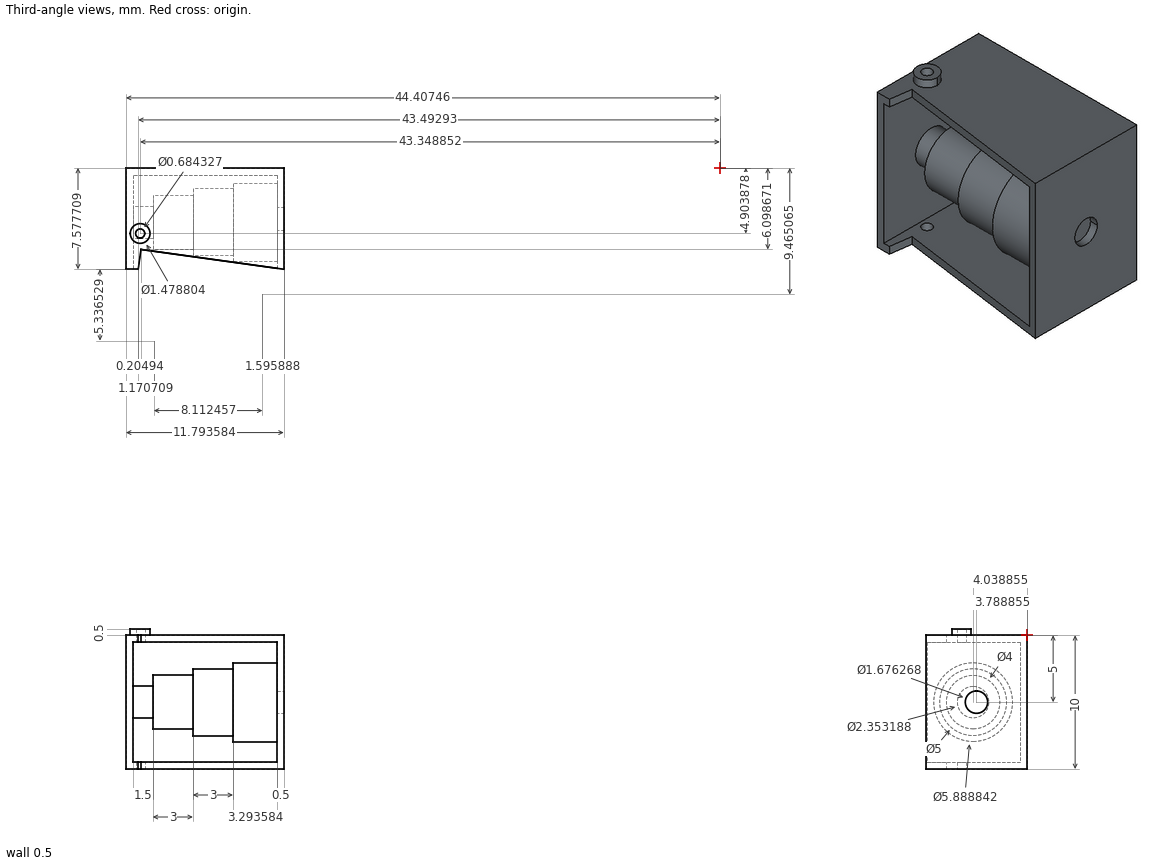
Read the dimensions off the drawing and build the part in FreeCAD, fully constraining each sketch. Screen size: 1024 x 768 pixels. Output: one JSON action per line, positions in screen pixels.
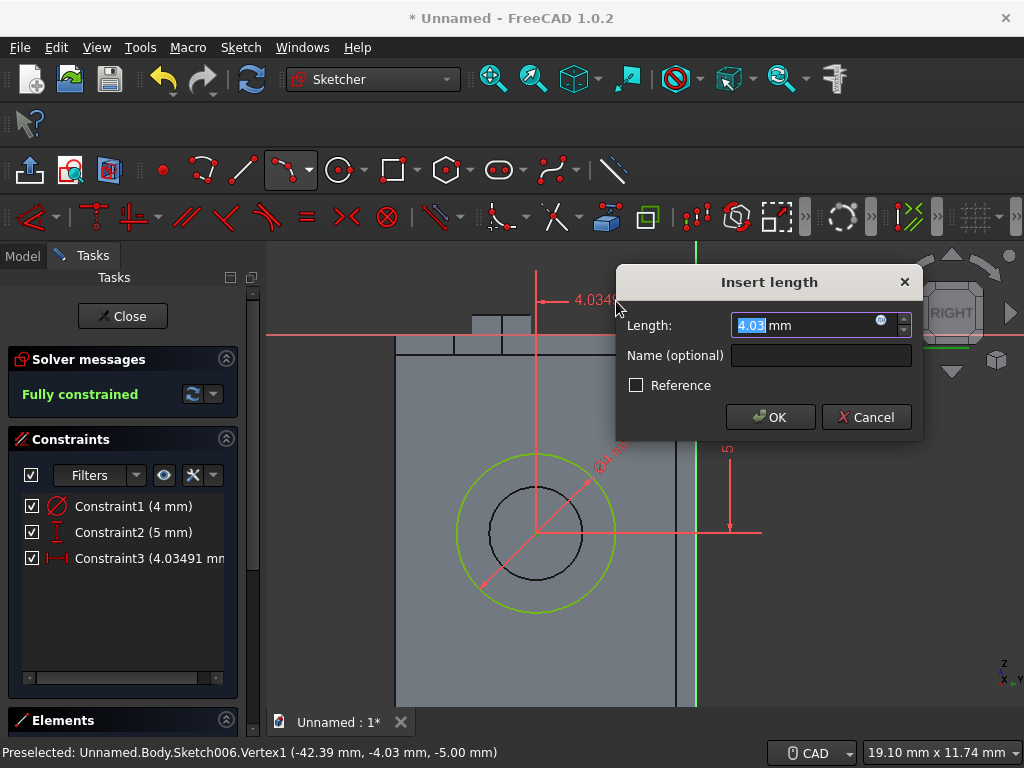
{"action": "type", "text": "4.038855"}
{"action": "key", "text": "Return"}
{"action": "key", "text": "Escape"}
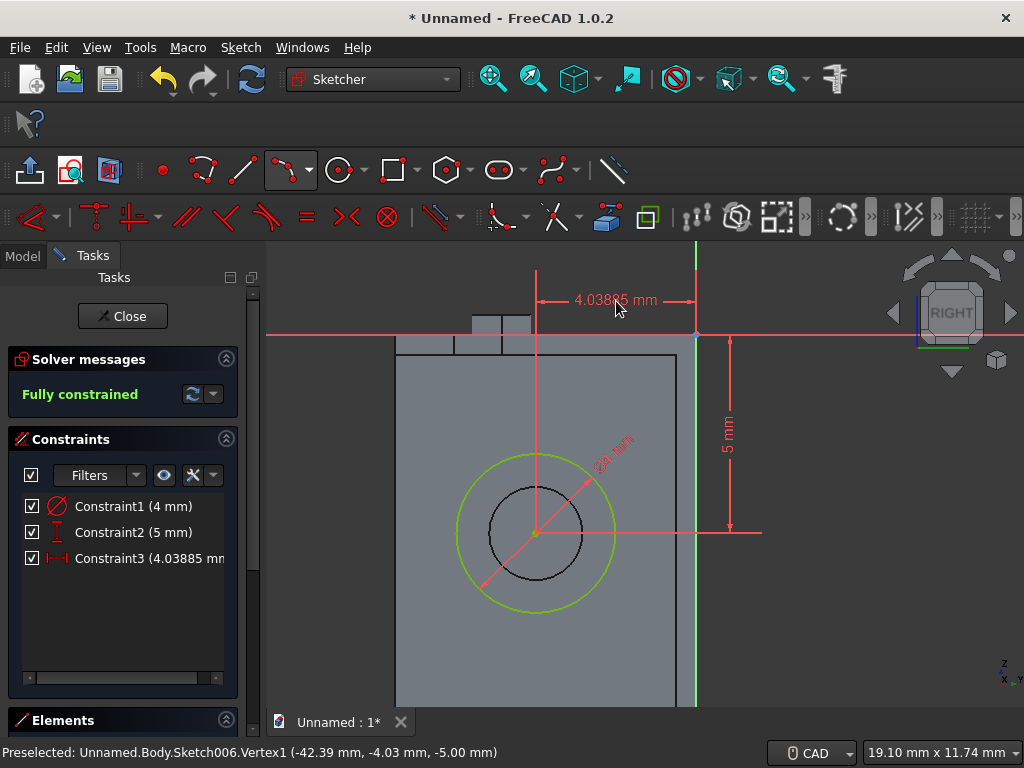
{"action": "left_click", "coordinate": [123, 316]}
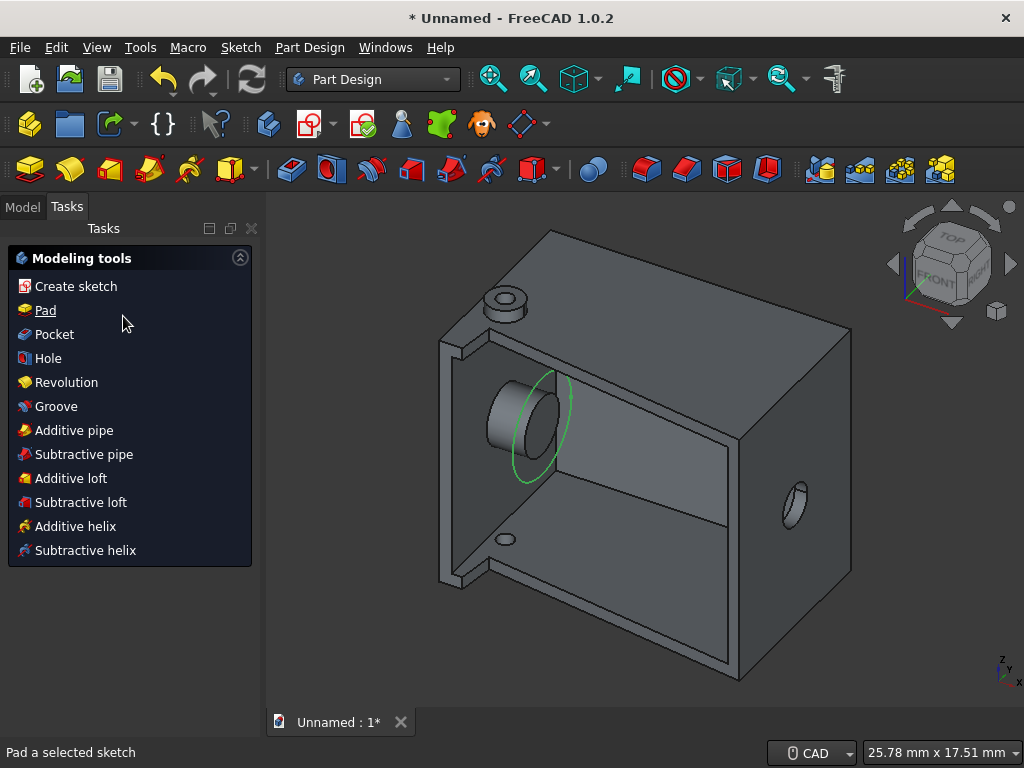
{"action": "left_click", "coordinate": [30, 170]}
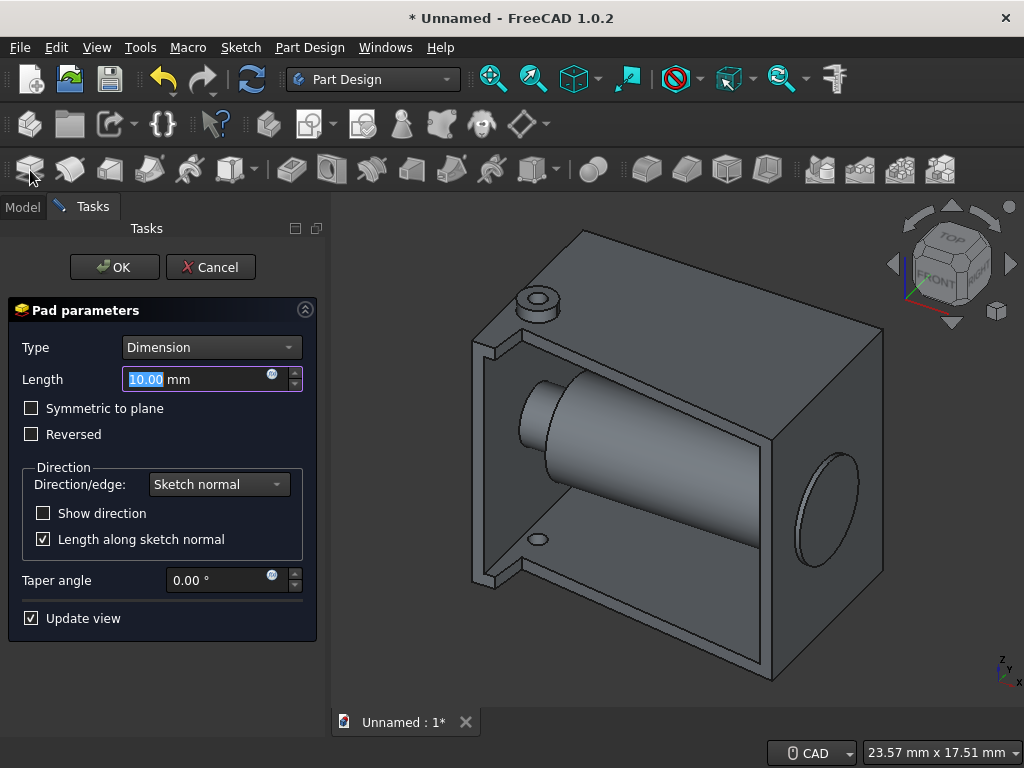
{"action": "type", "text": "3"}
{"action": "key", "text": "Tab"}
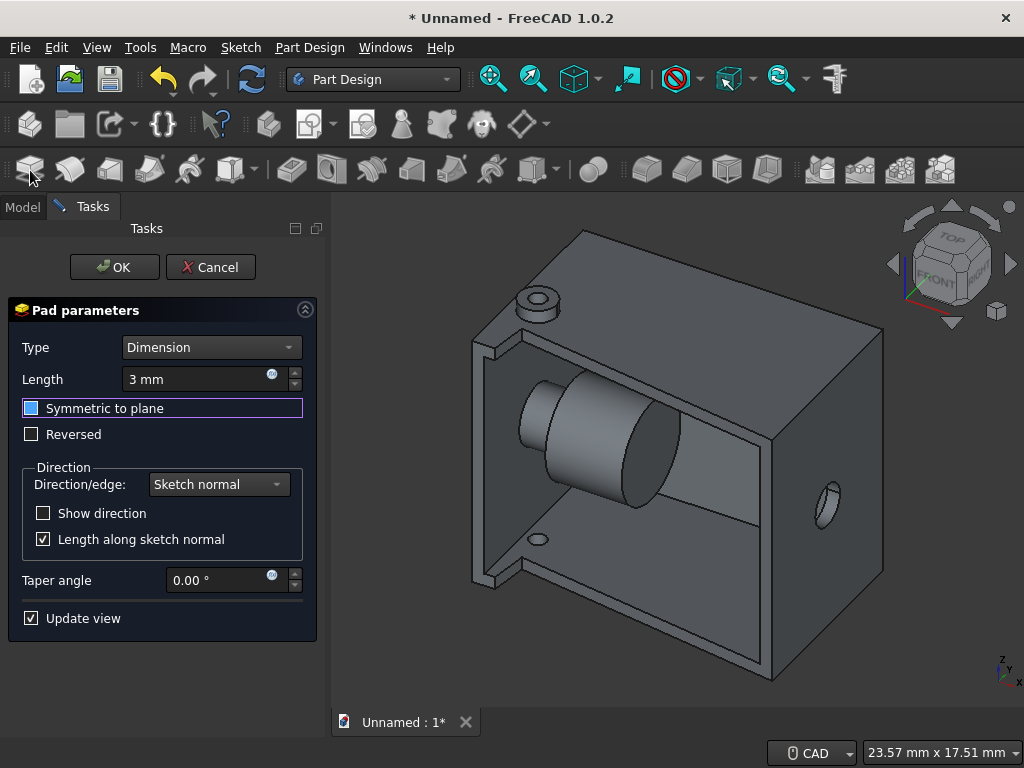
{"action": "left_click", "coordinate": [115, 267]}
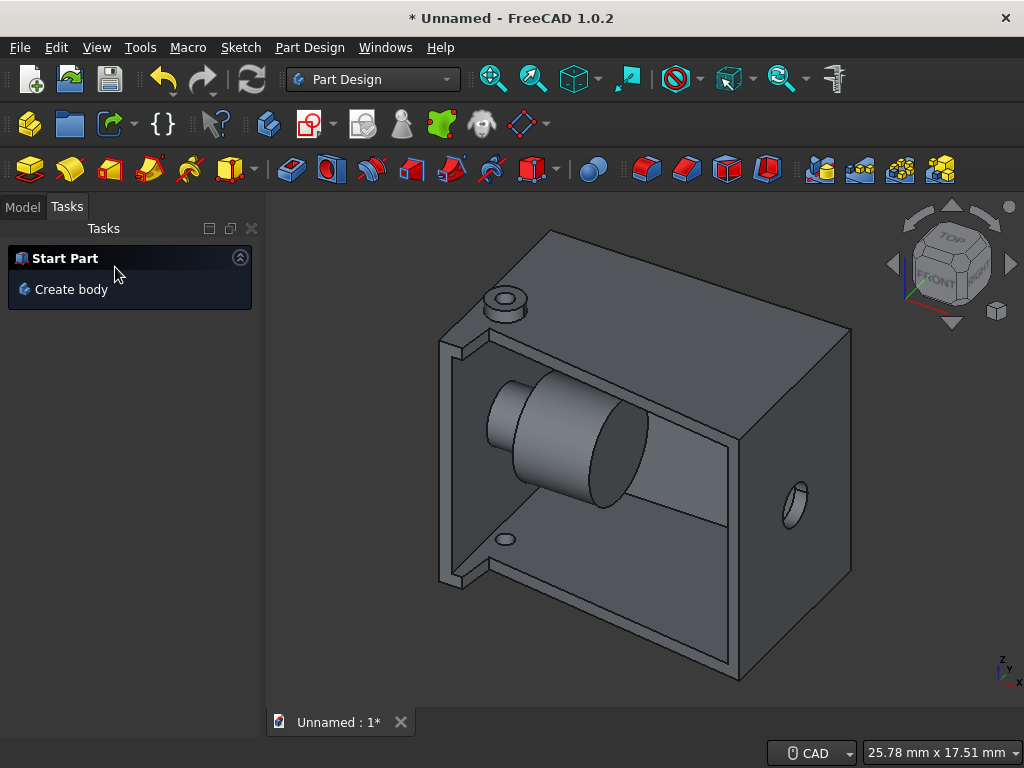
{"action": "left_click", "coordinate": [619, 451]}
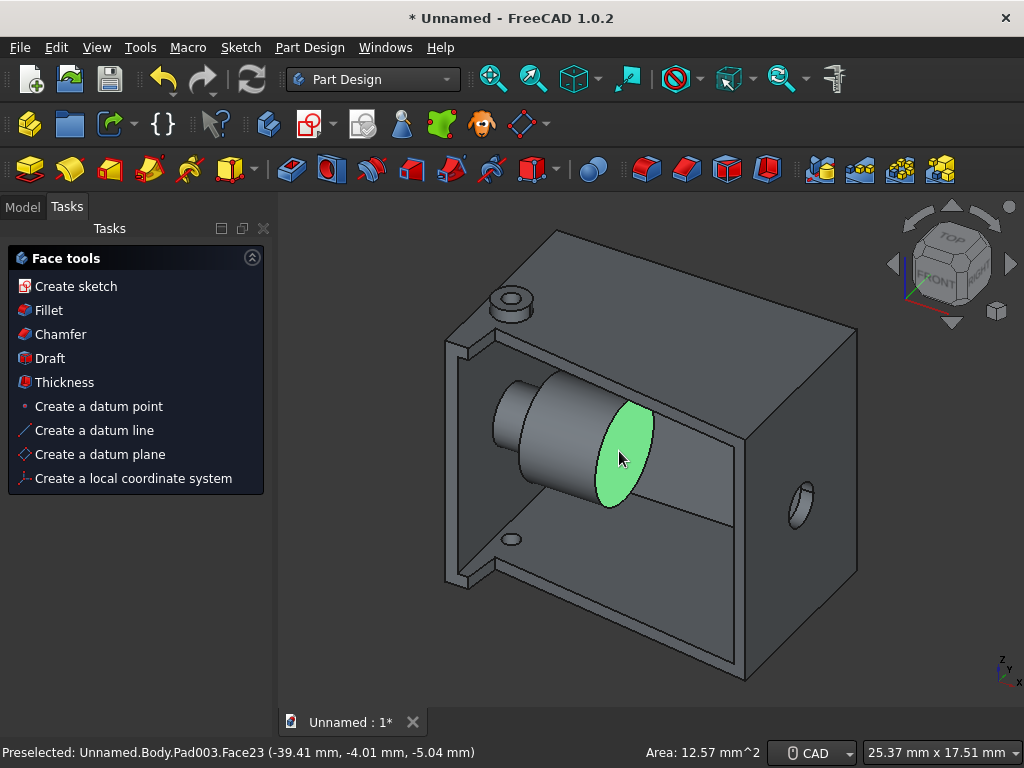
{"action": "left_click", "coordinate": [310, 124]}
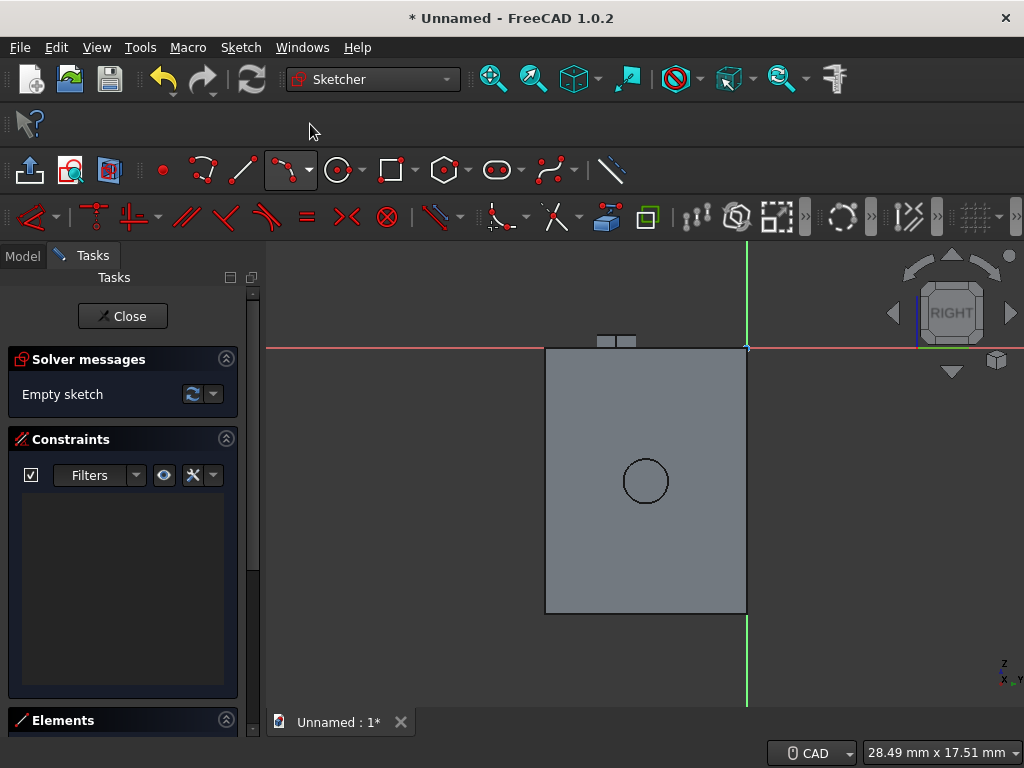
{"action": "scroll", "coordinate": [829, 395], "scroll_direction": "up", "scroll_amount": 2}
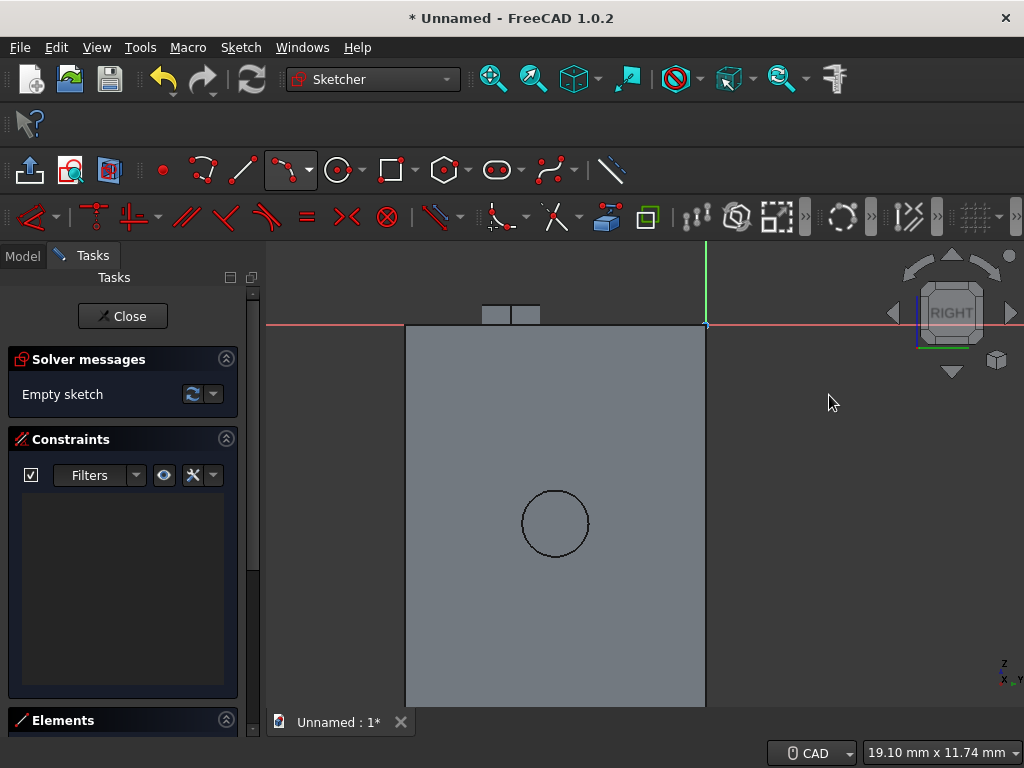
{"action": "left_click", "coordinate": [338, 170]}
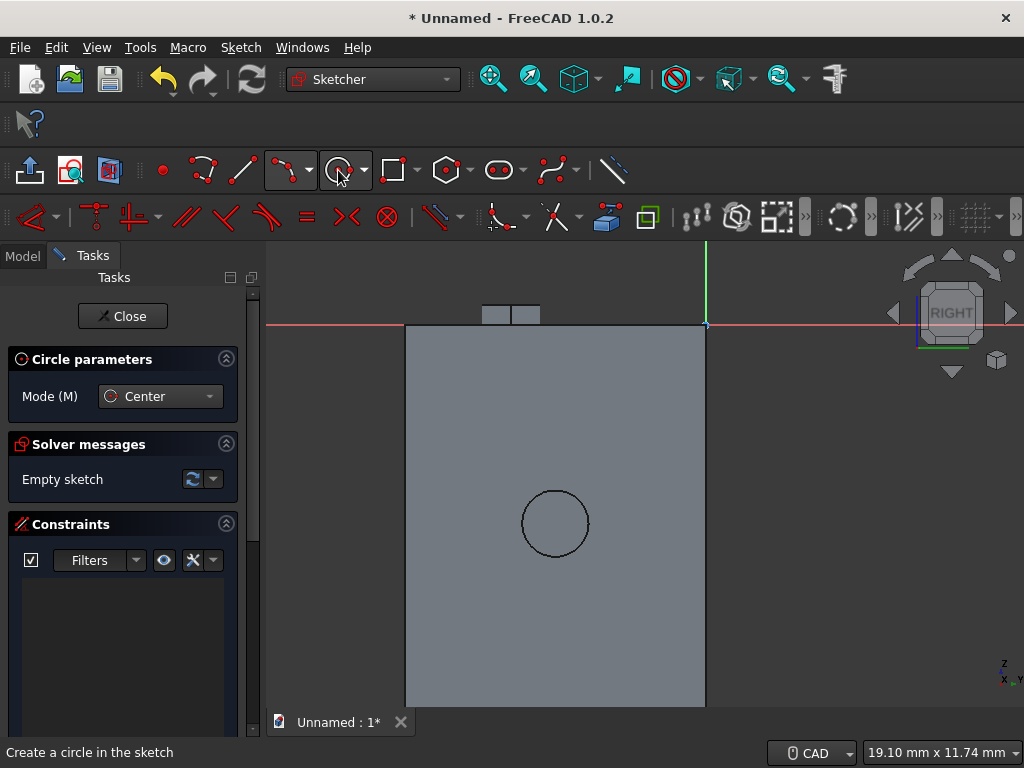
{"action": "left_click", "coordinate": [545, 524]}
{"action": "left_click", "coordinate": [616, 453]}
{"action": "key", "text": "Escape"}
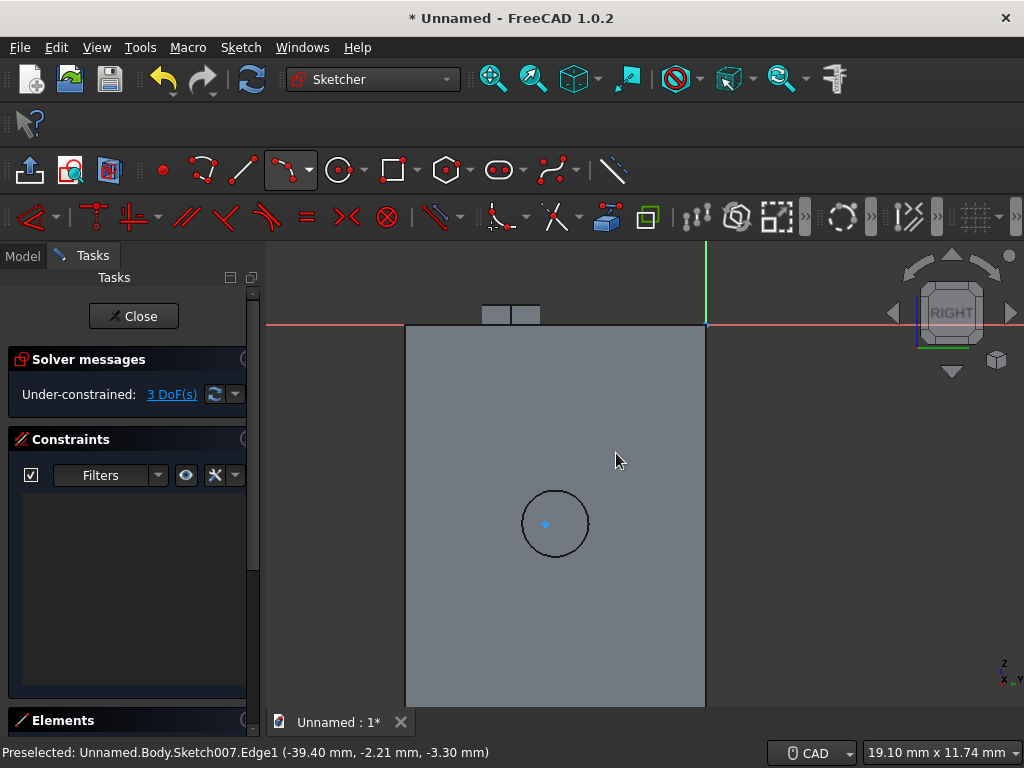
{"action": "left_click", "coordinate": [32, 218]}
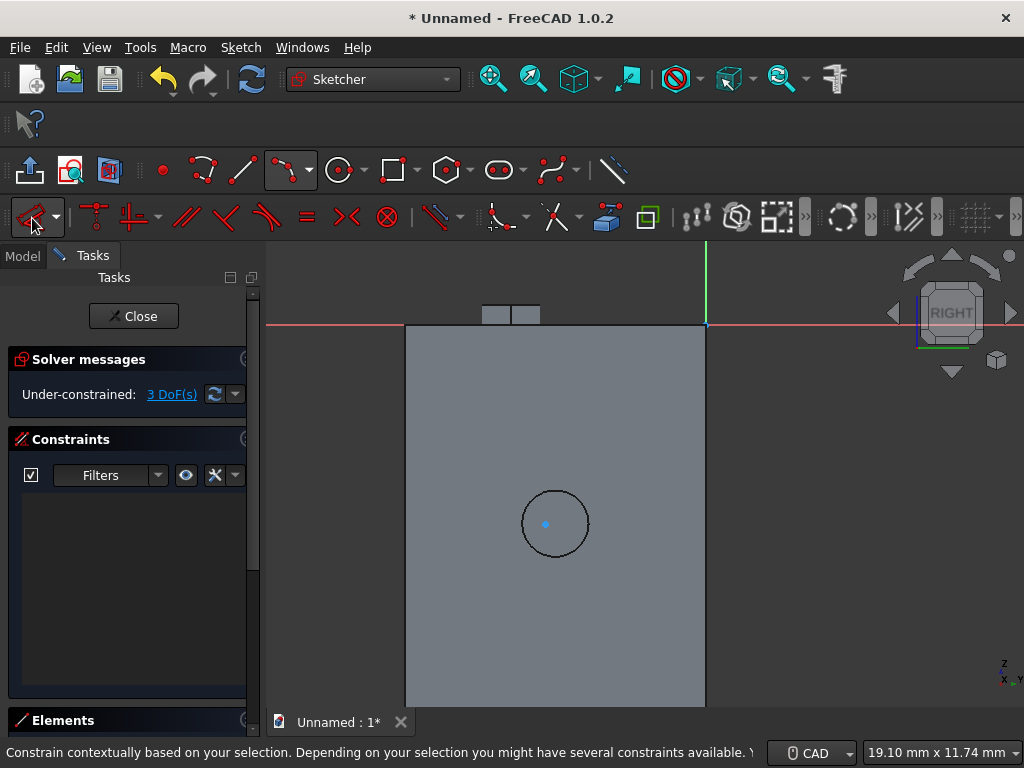
{"action": "left_click", "coordinate": [616, 454]}
{"action": "left_click", "coordinate": [639, 431]}